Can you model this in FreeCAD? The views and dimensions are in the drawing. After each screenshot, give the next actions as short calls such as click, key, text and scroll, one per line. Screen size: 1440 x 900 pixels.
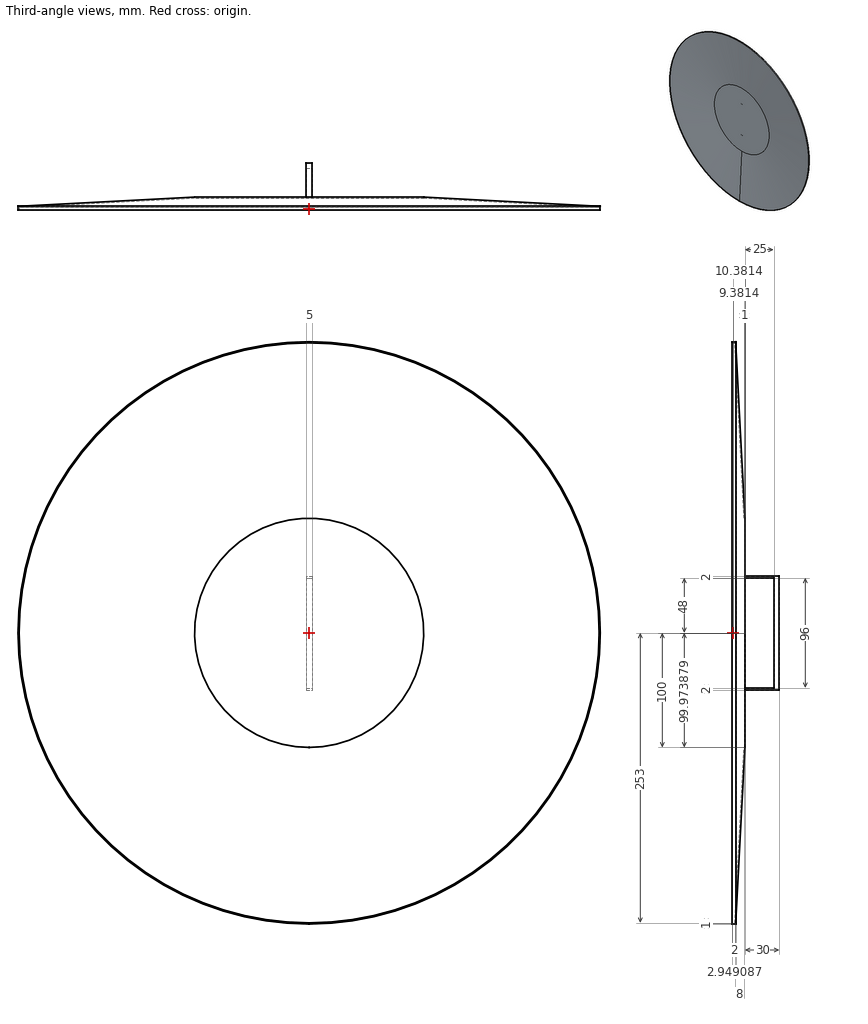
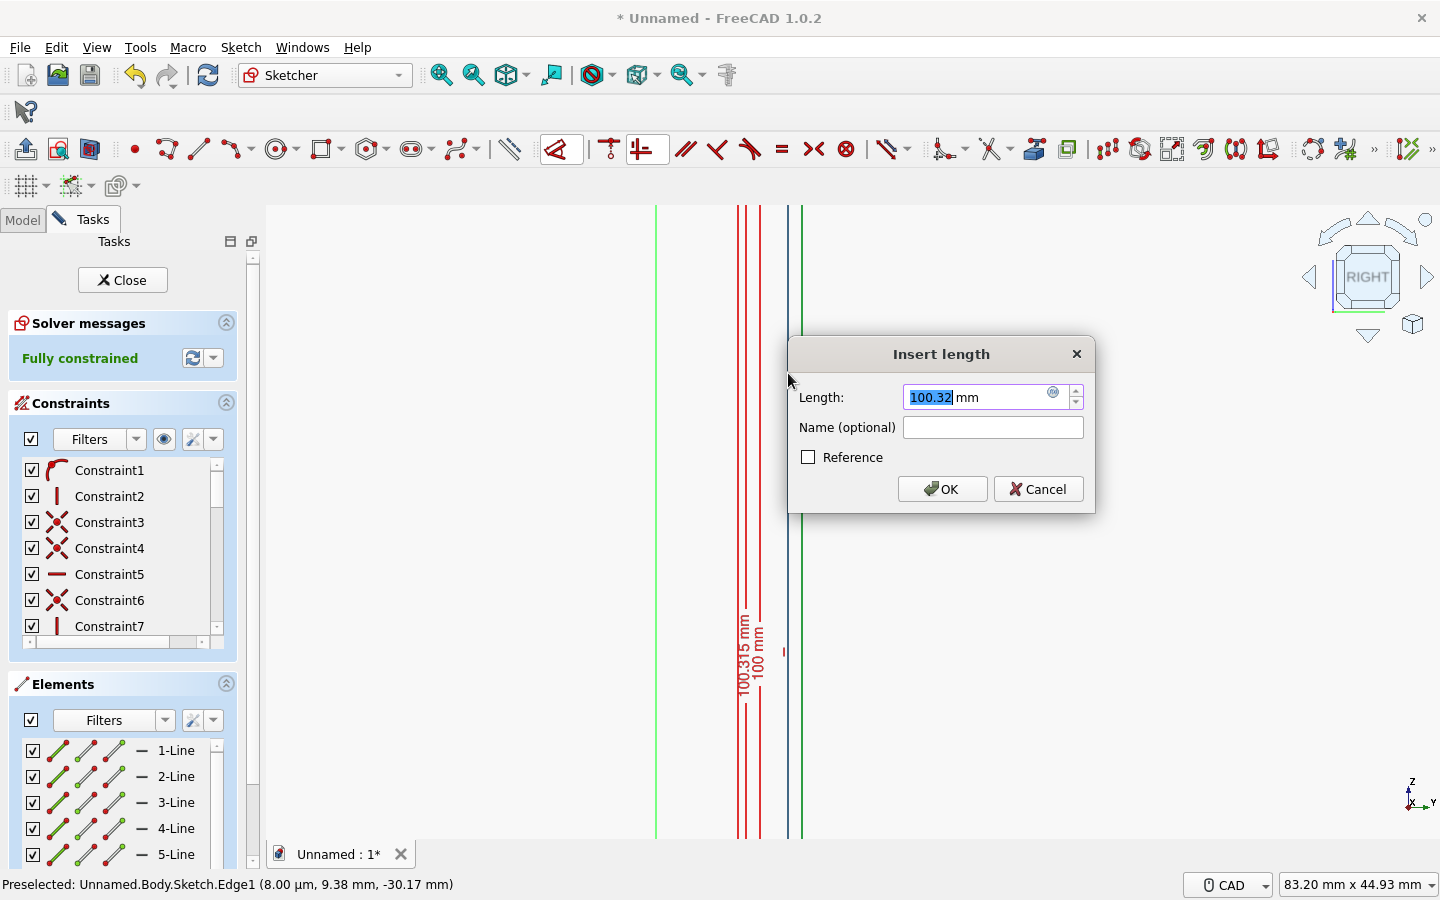
text(99.973879)
key(Return)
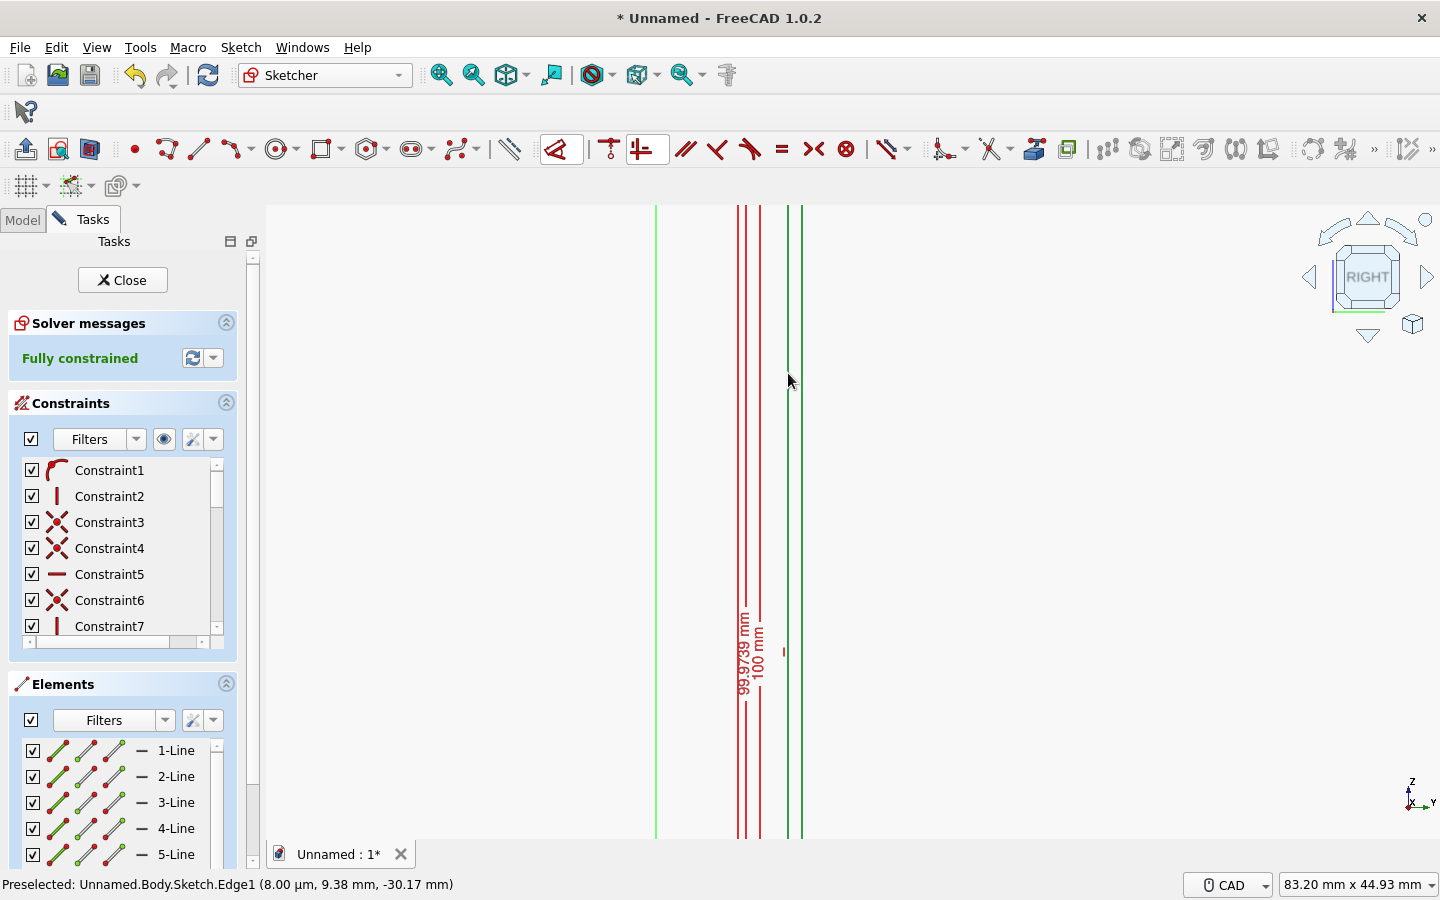
click(123, 280)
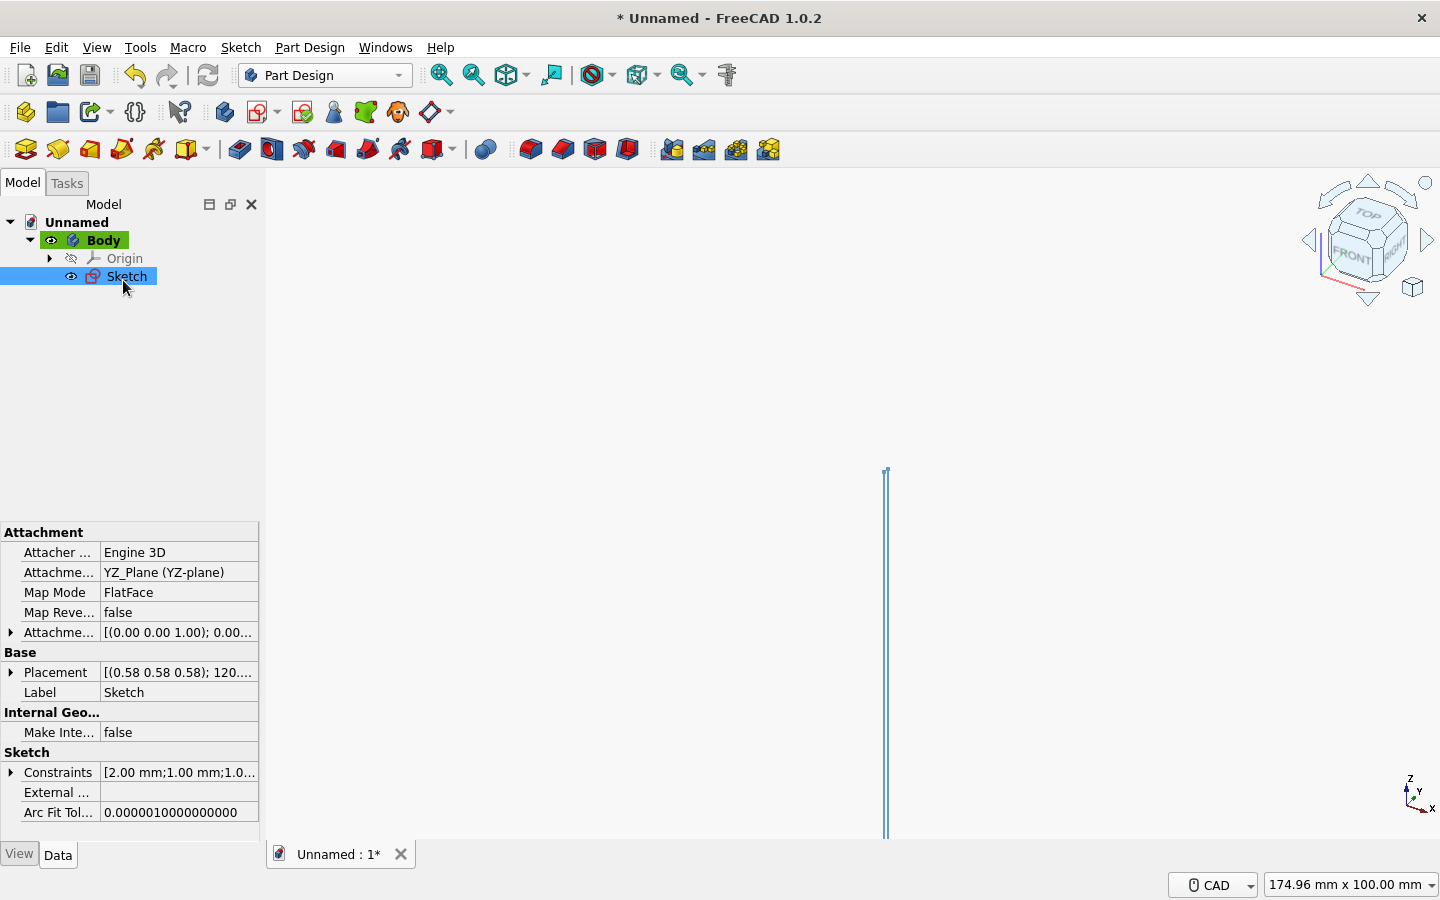
click(58, 150)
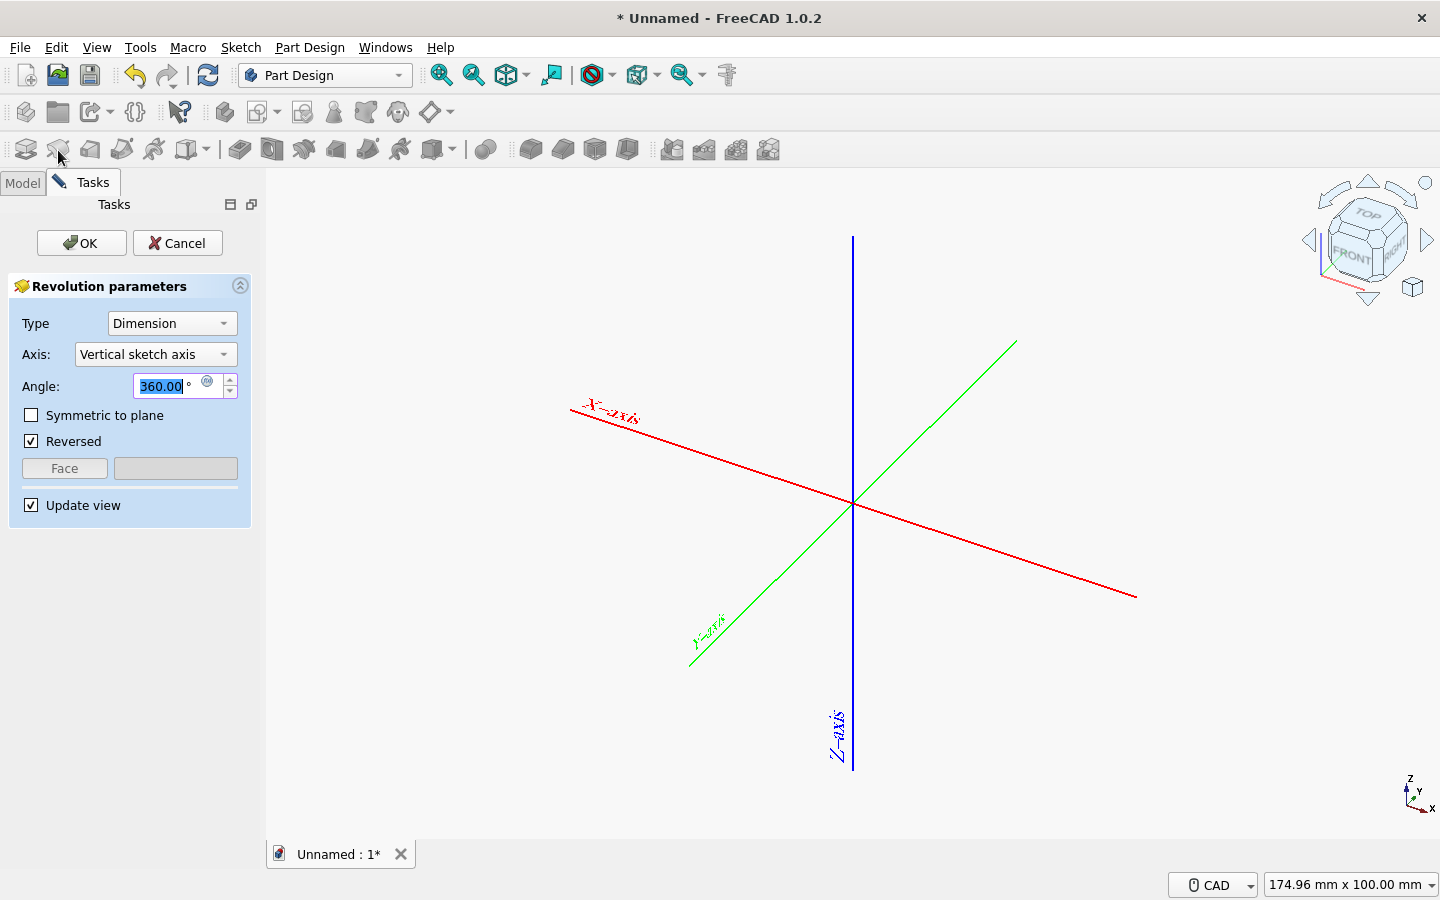
click(156, 354)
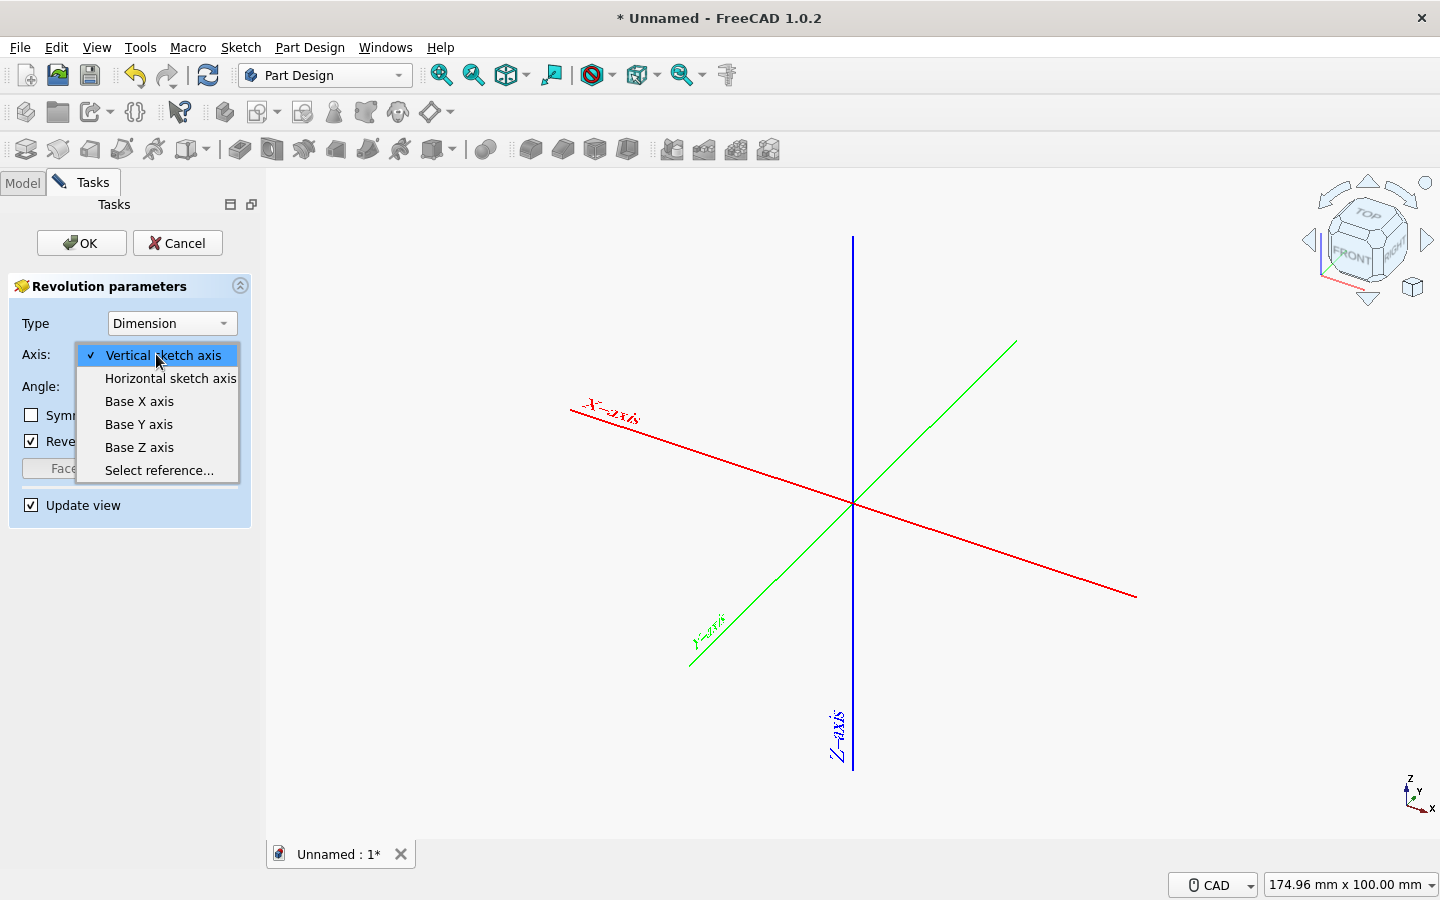
click(156, 378)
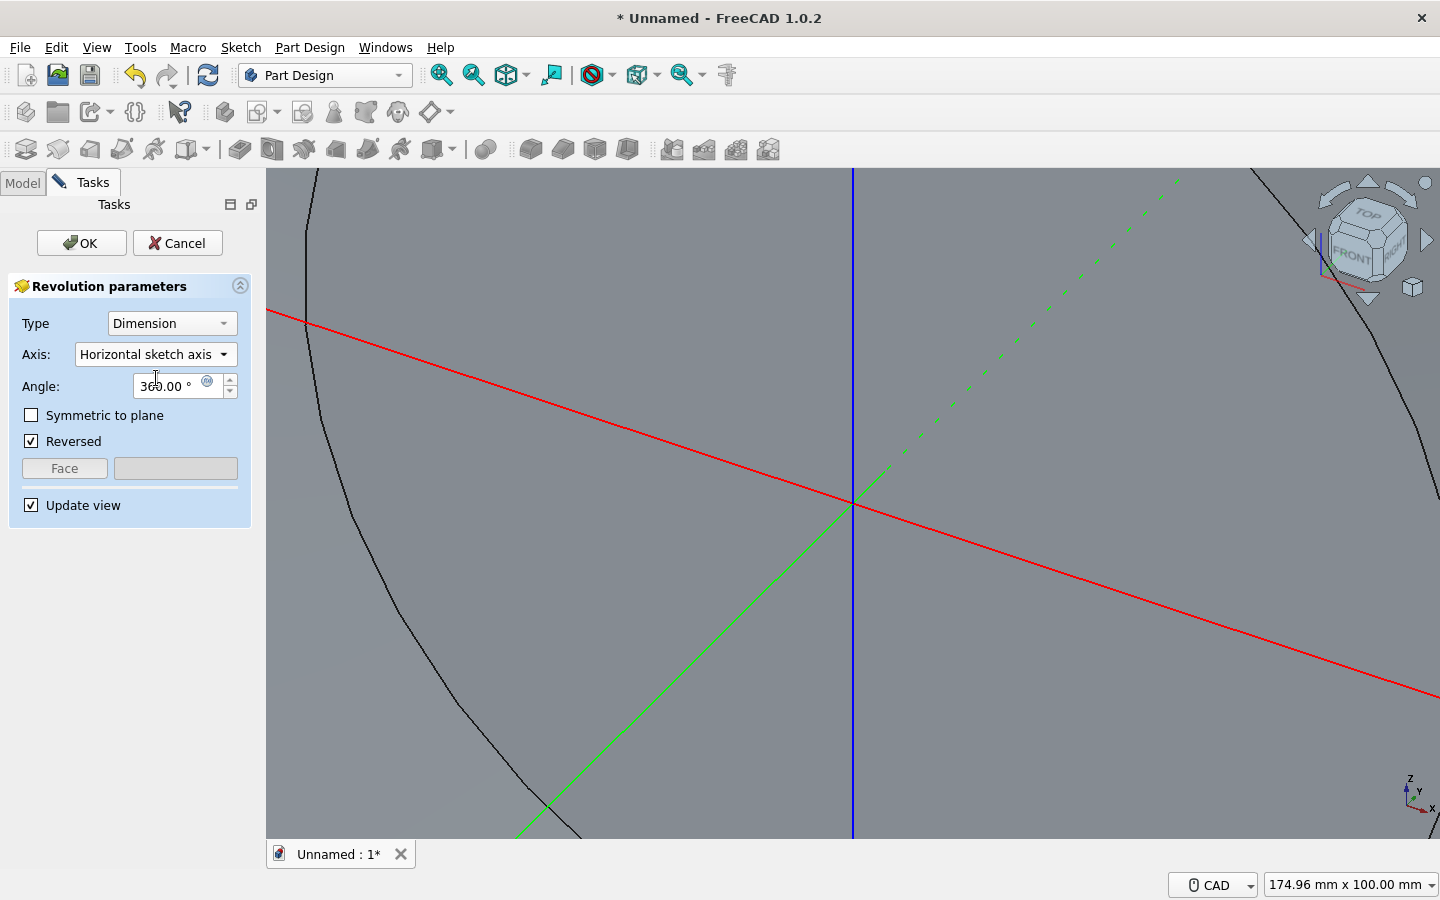
click(82, 243)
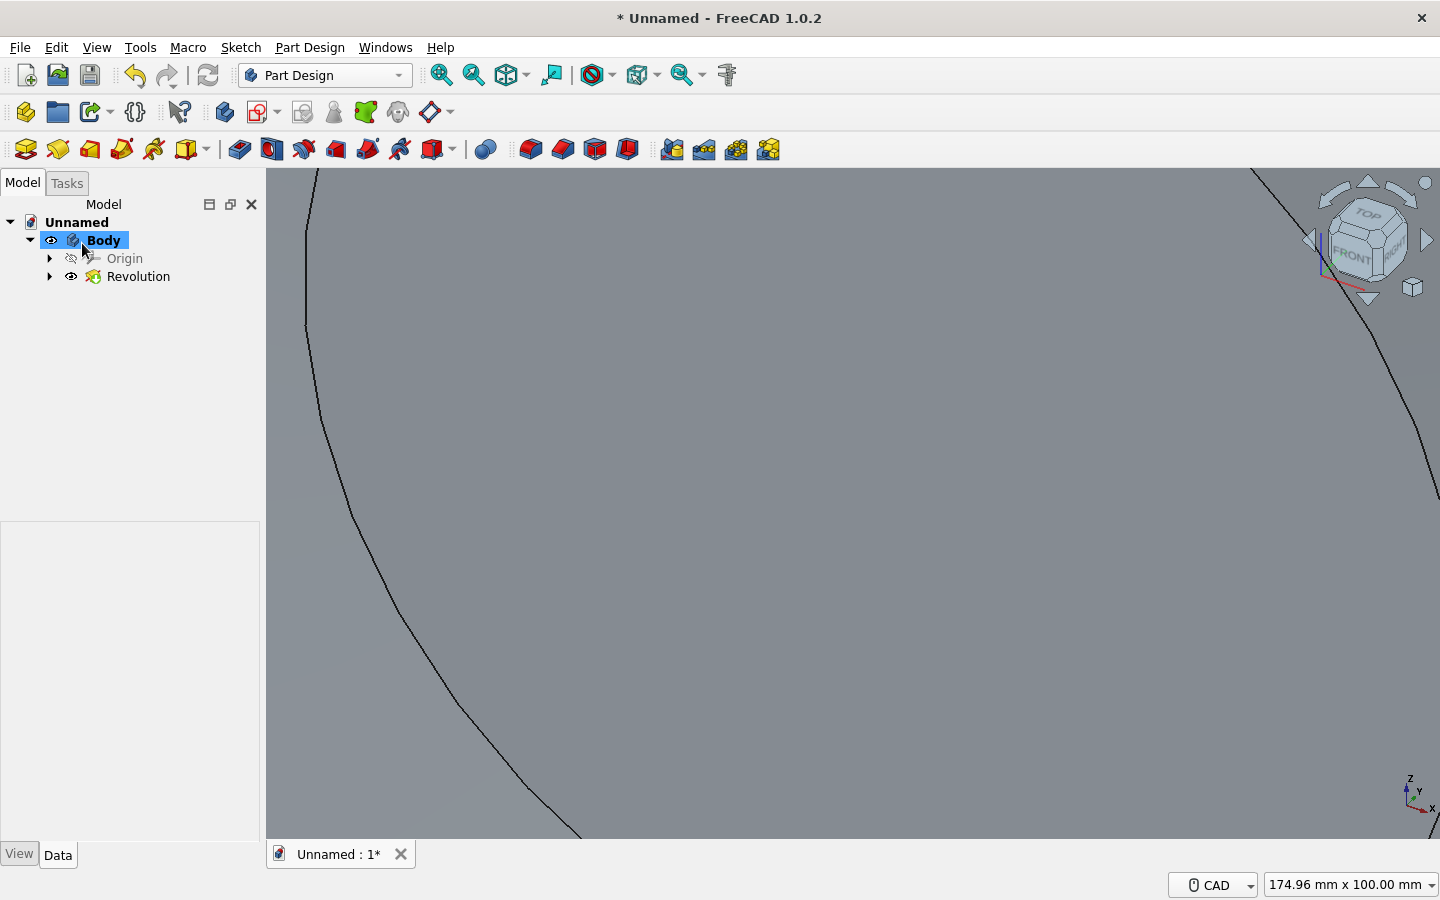
key(v)
key(f)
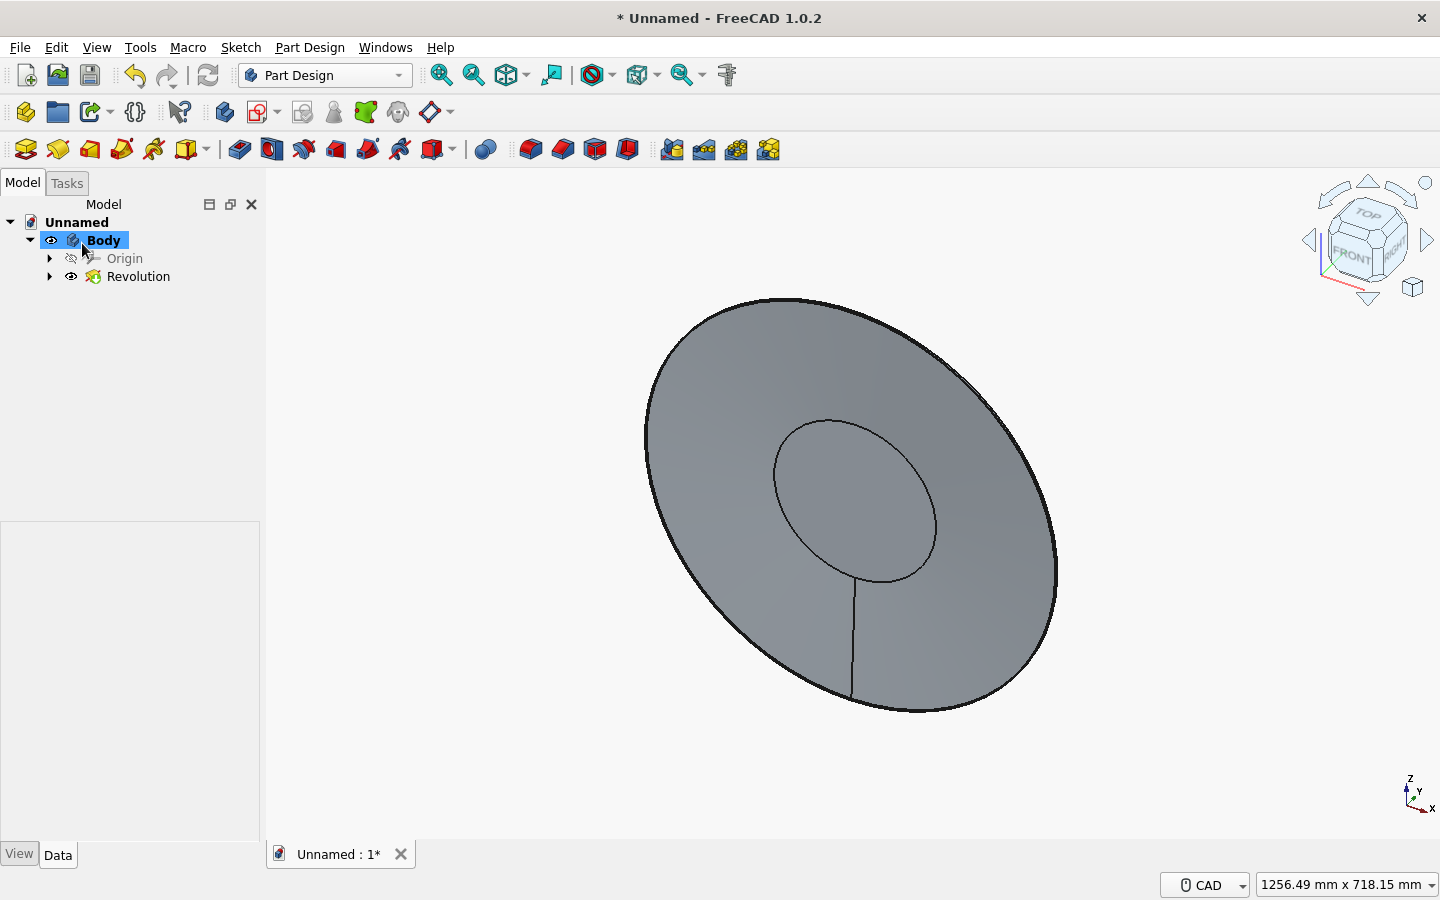
click(258, 112)